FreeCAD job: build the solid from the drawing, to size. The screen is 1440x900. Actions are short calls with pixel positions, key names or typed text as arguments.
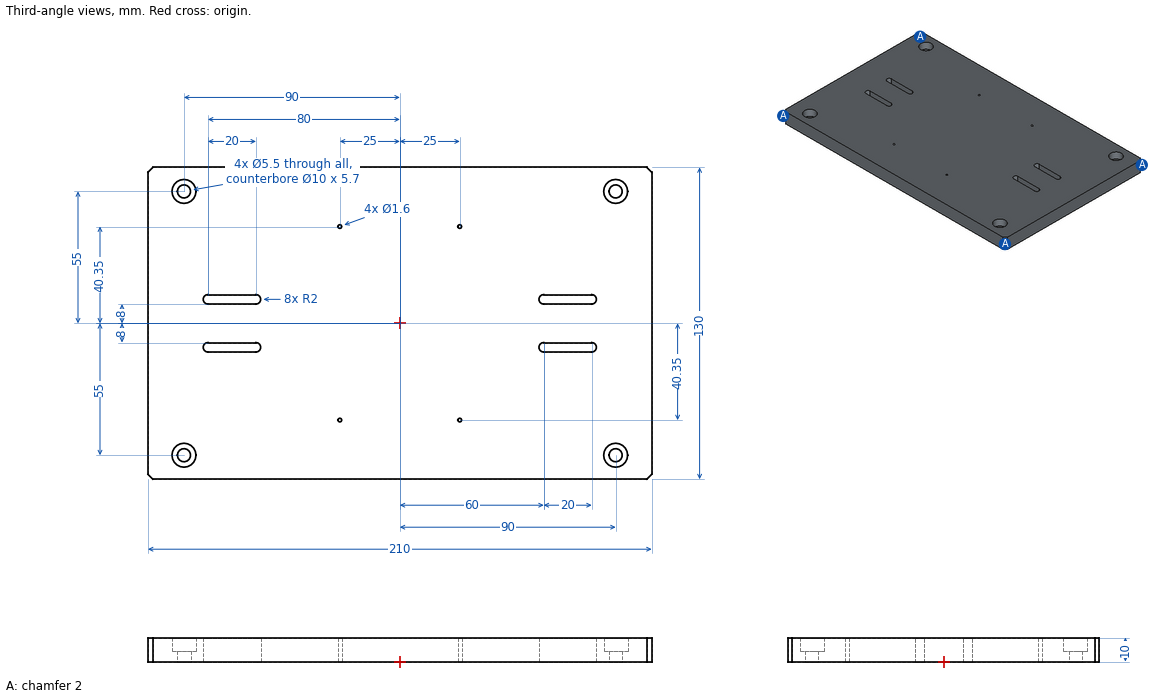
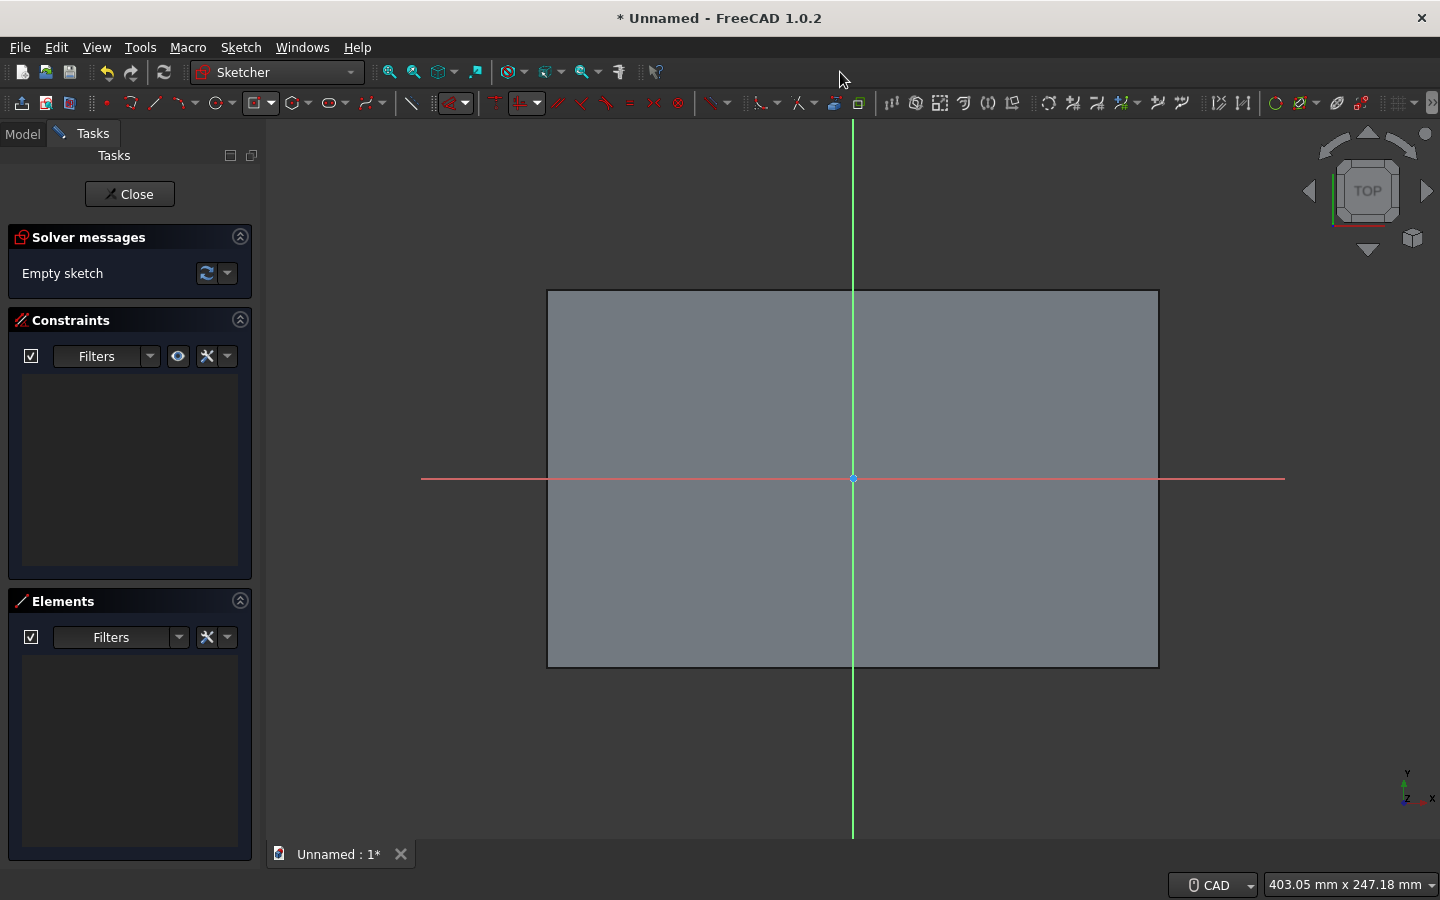
scroll(992, 479, up, 2)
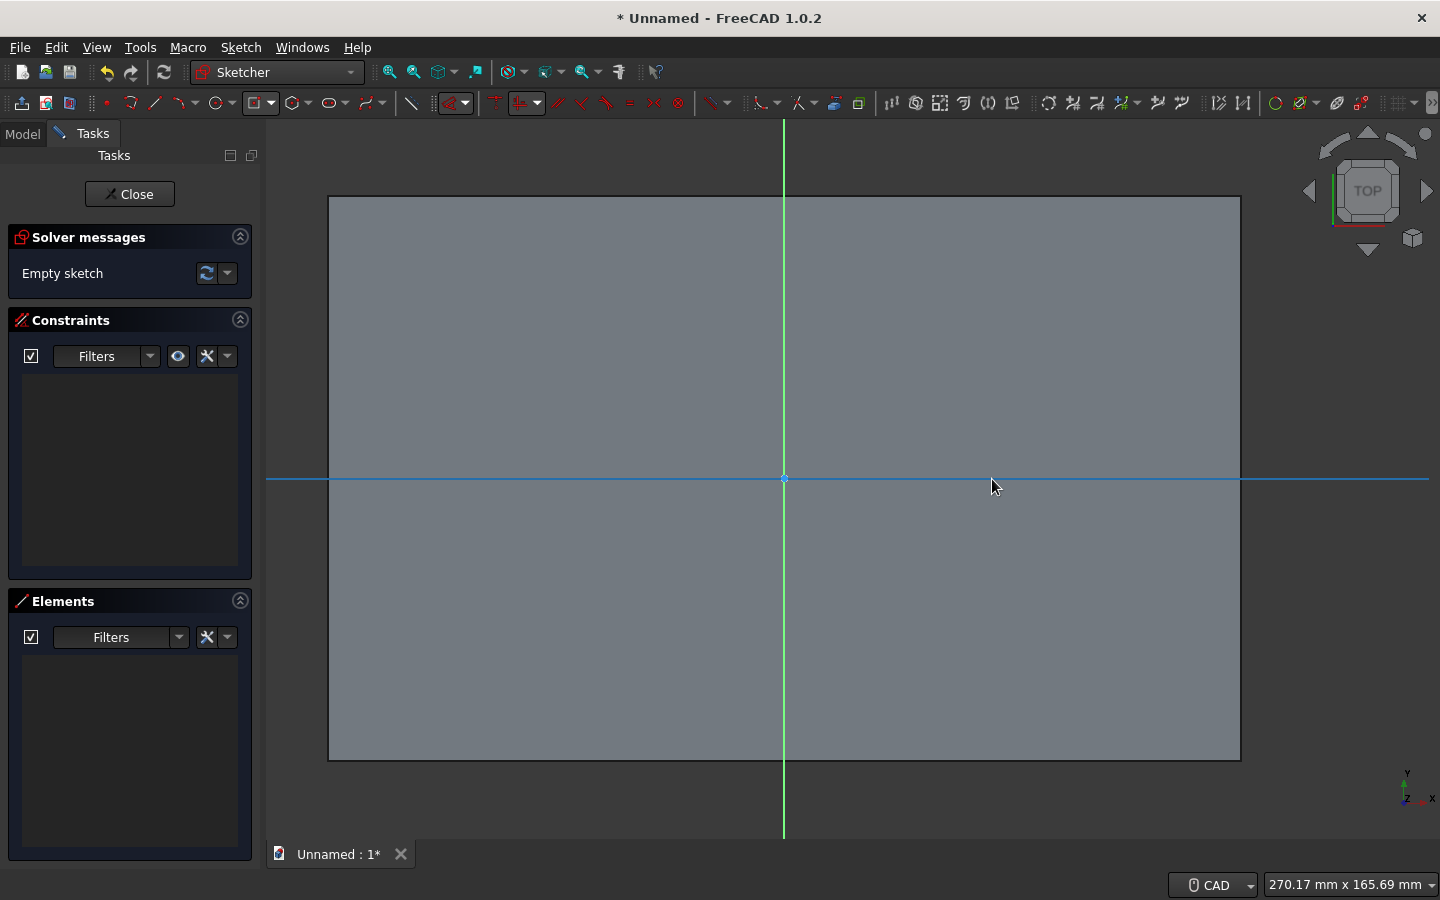
click(330, 104)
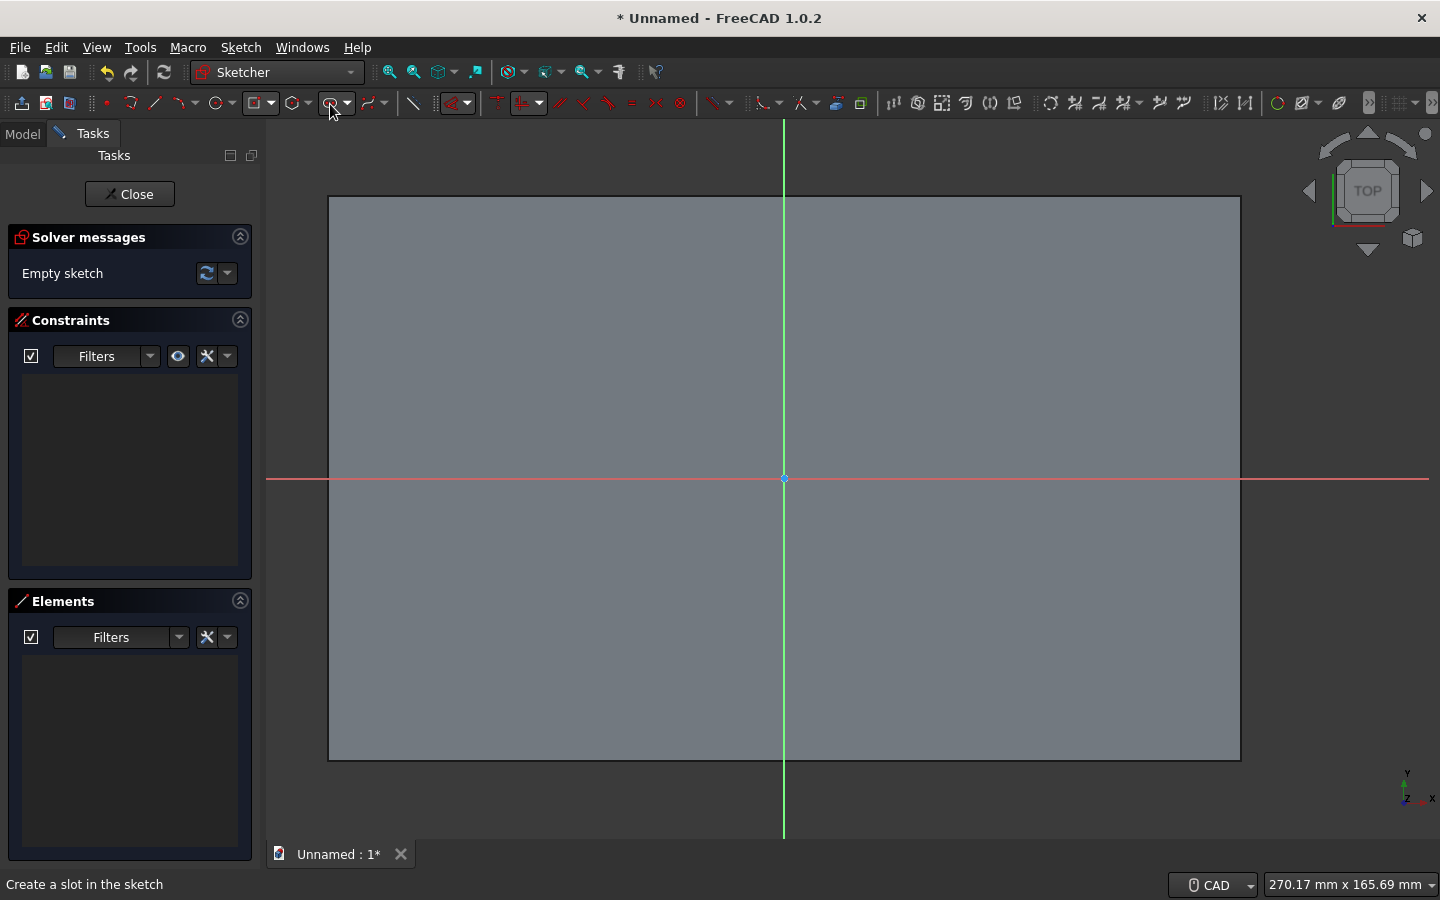
scroll(437, 435, up, 5)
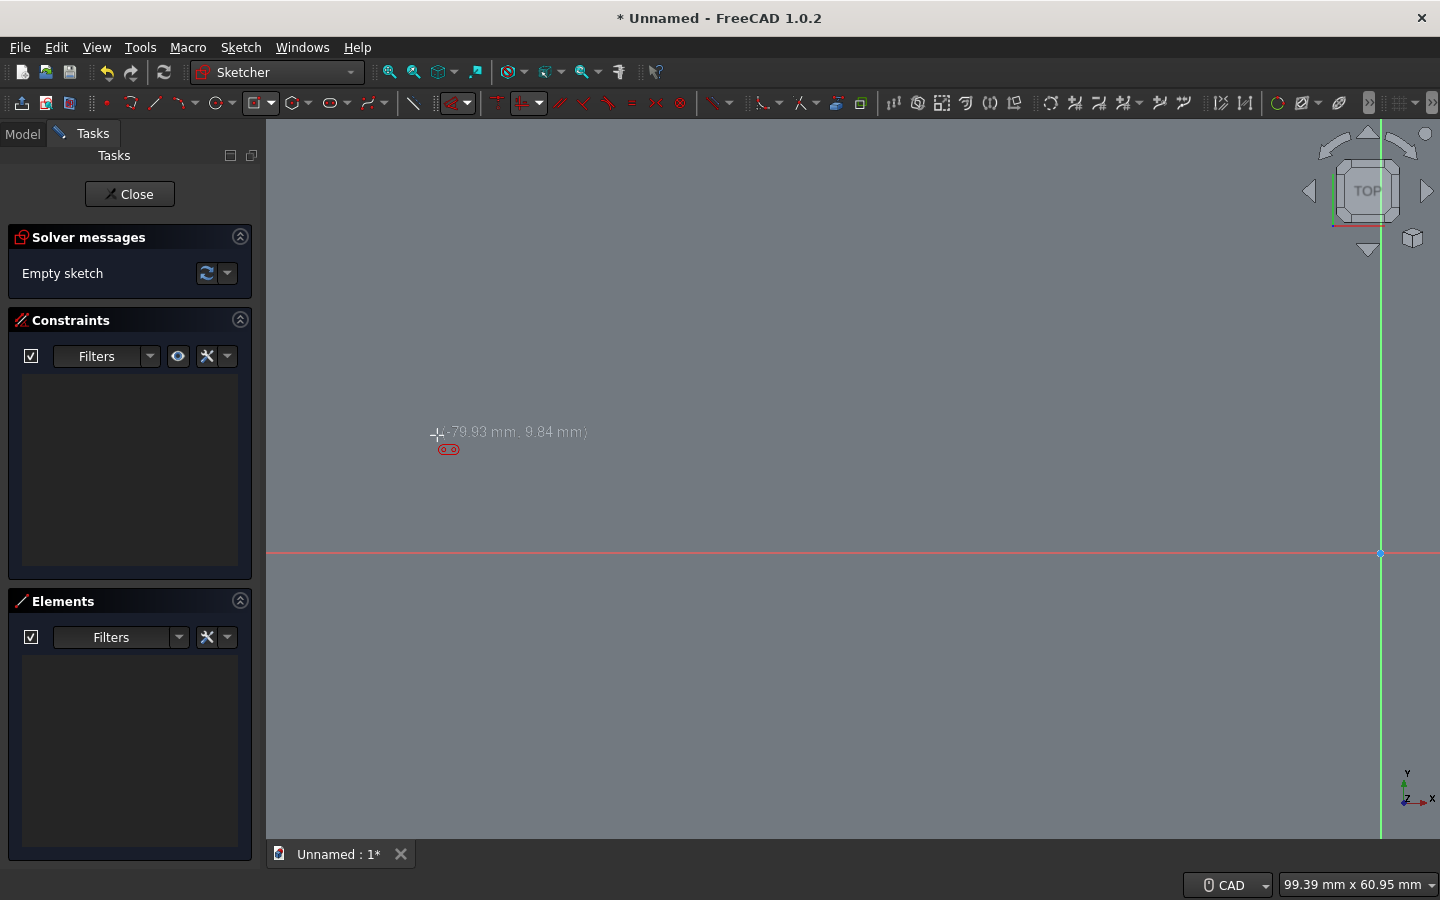
click(436, 435)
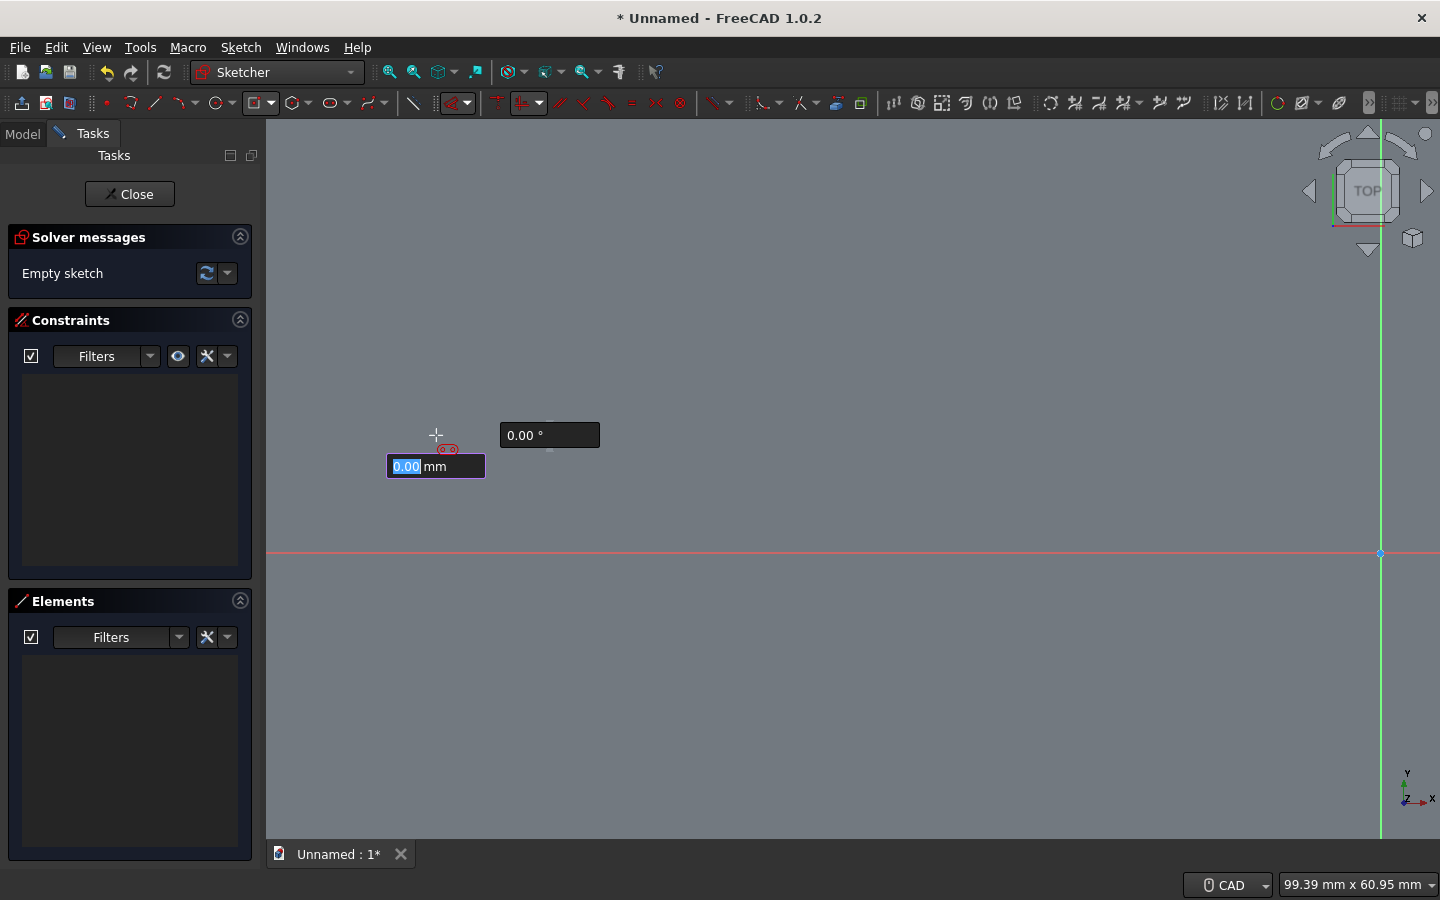
click(672, 435)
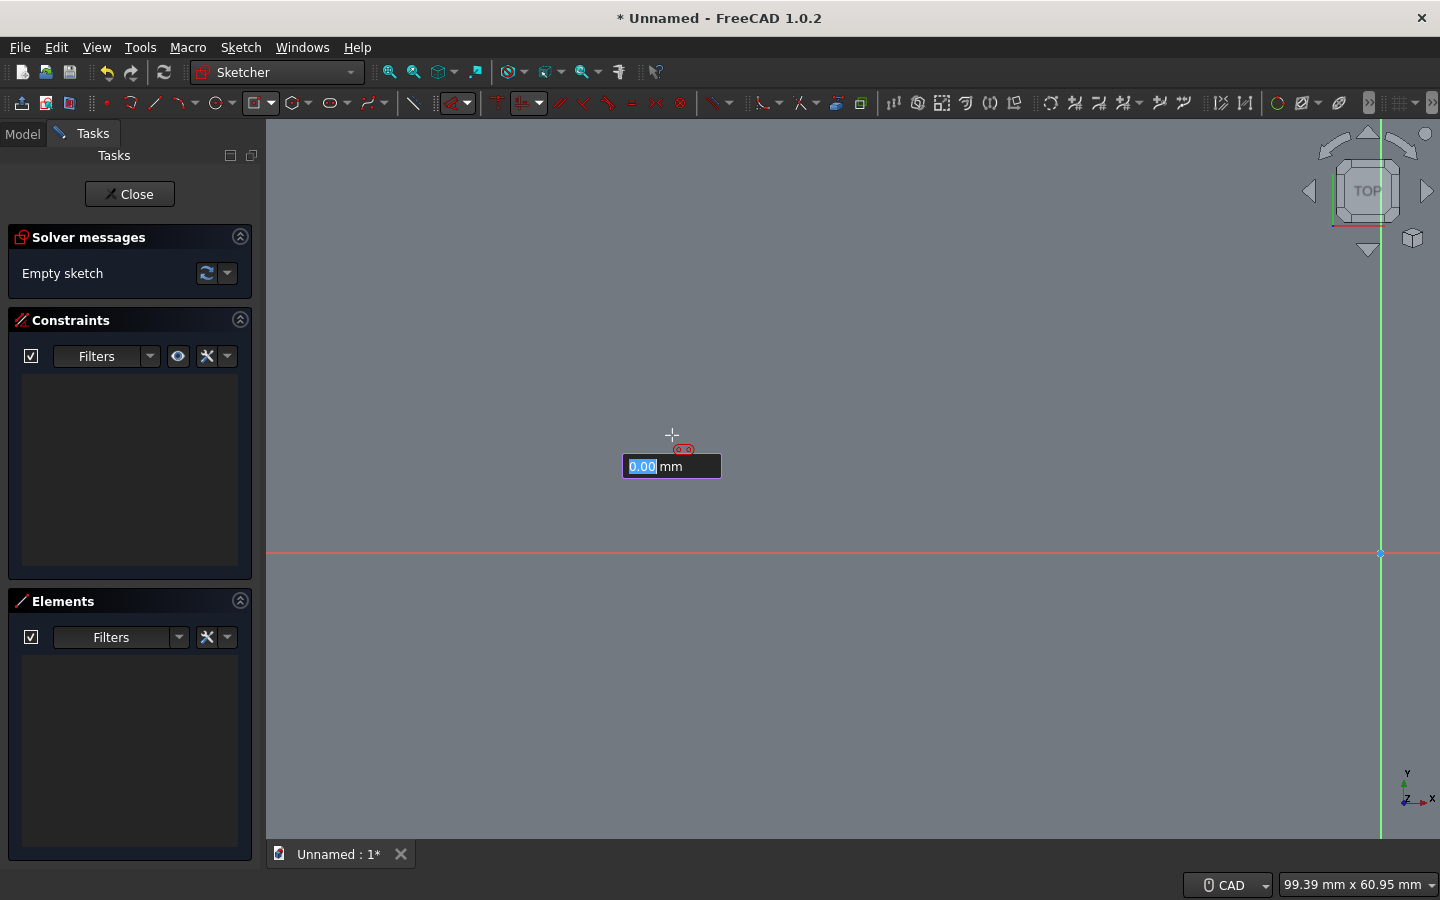
click(554, 459)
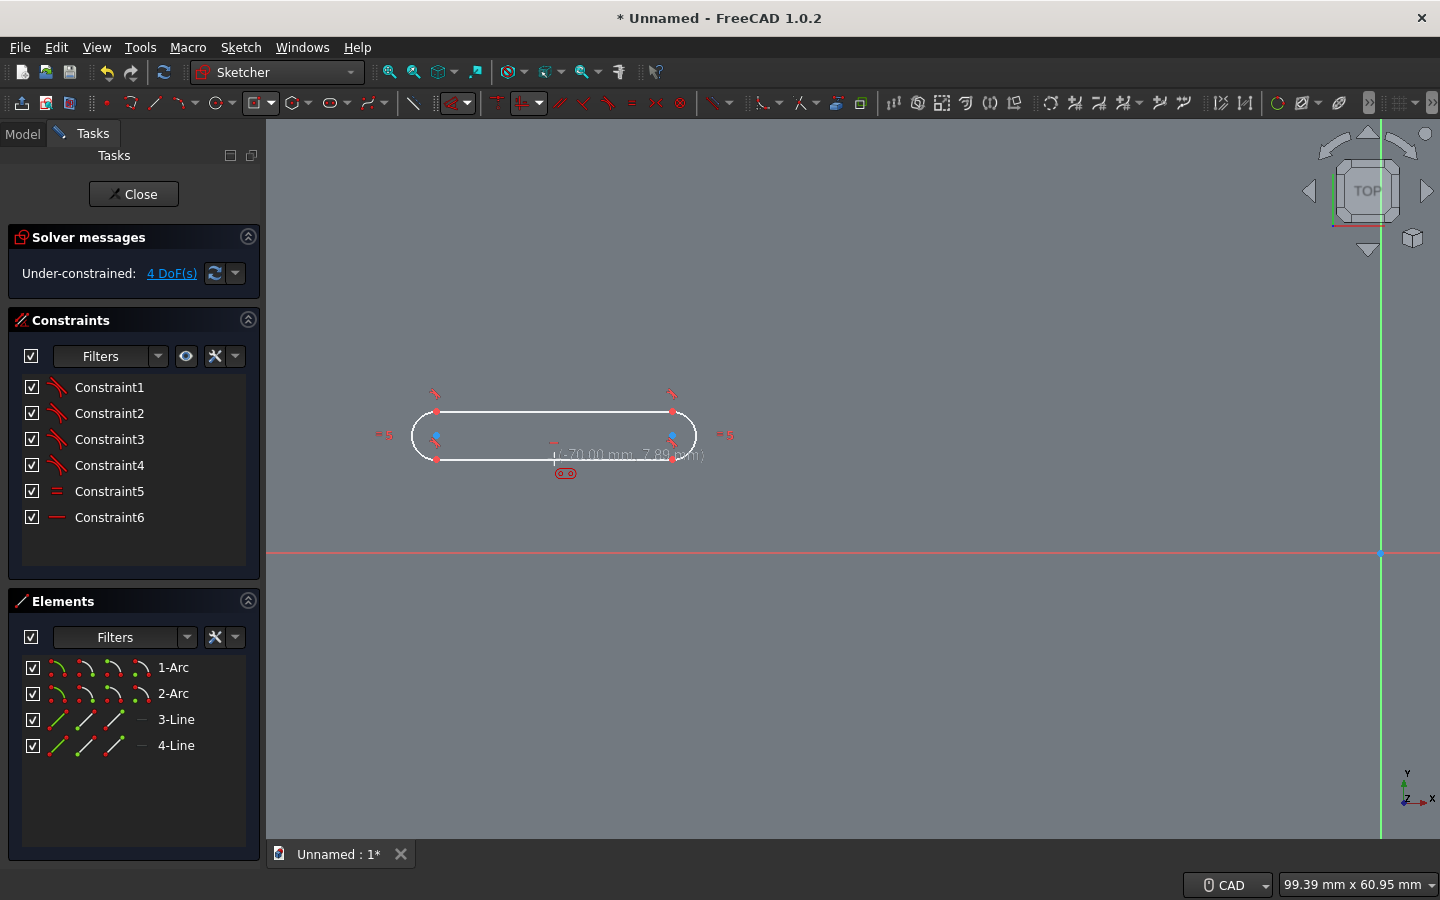
click(436, 671)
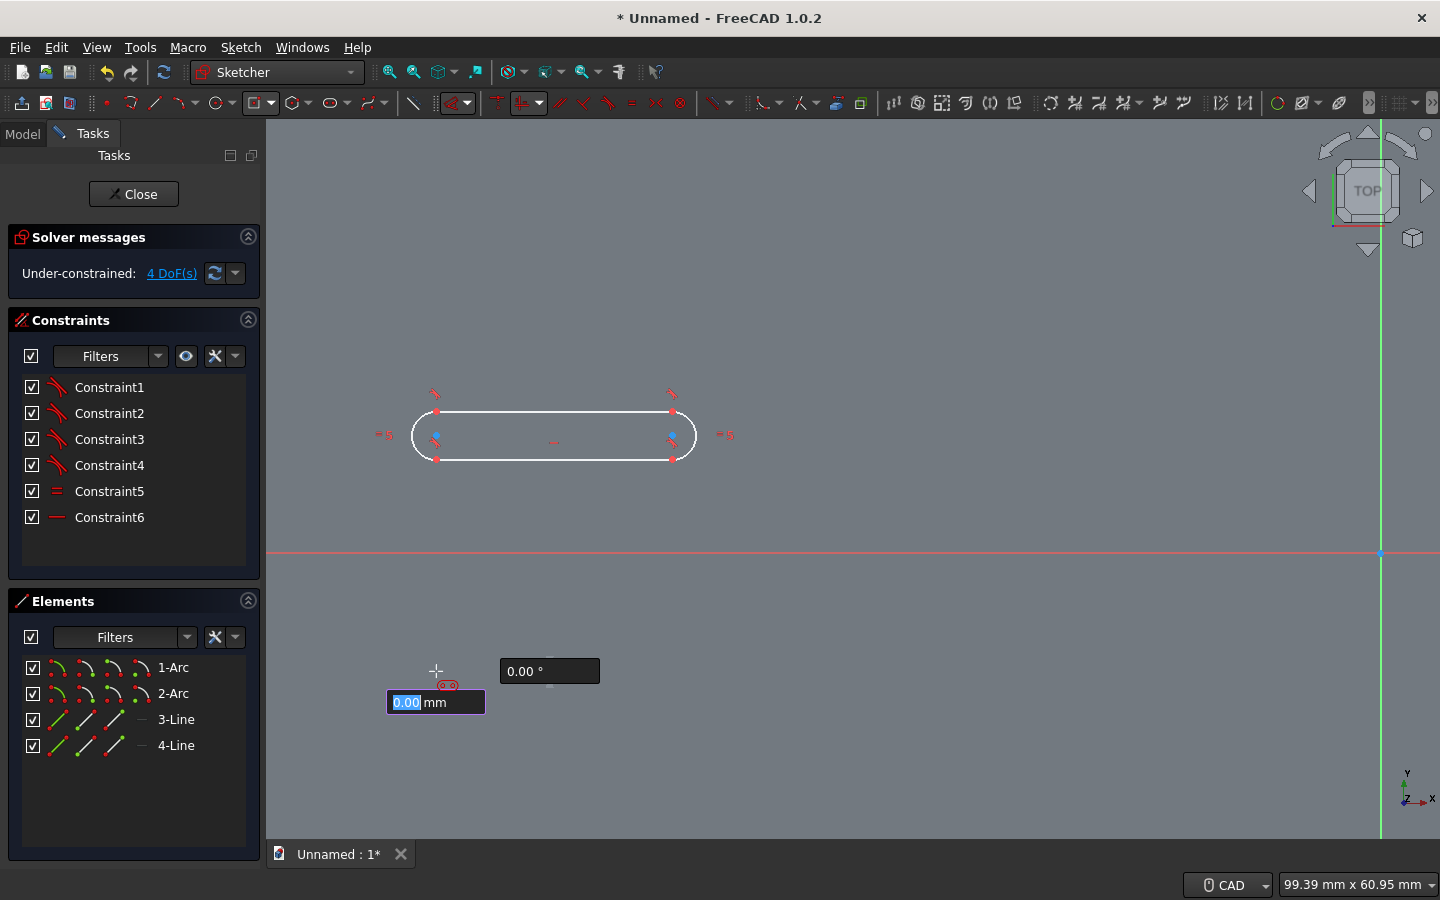
click(672, 671)